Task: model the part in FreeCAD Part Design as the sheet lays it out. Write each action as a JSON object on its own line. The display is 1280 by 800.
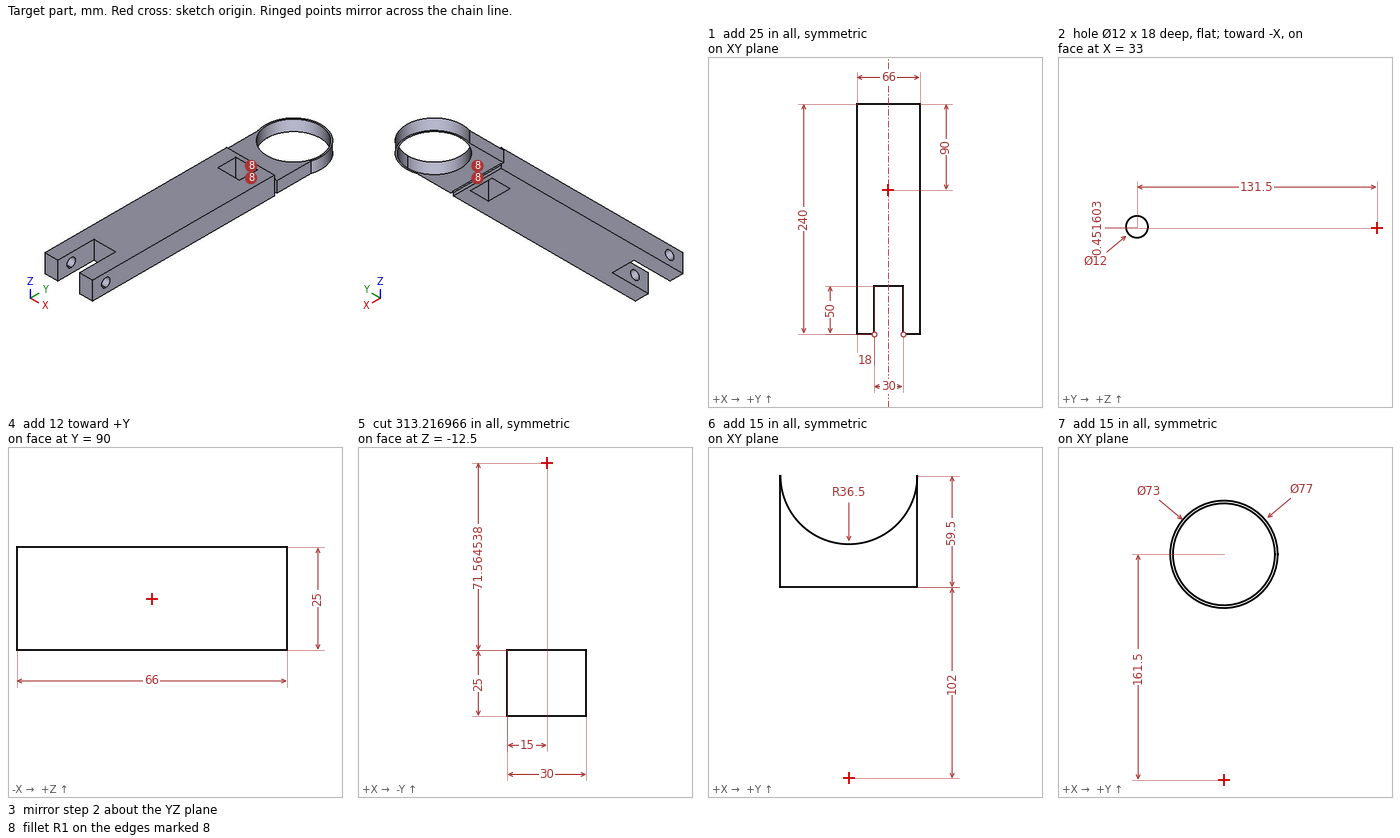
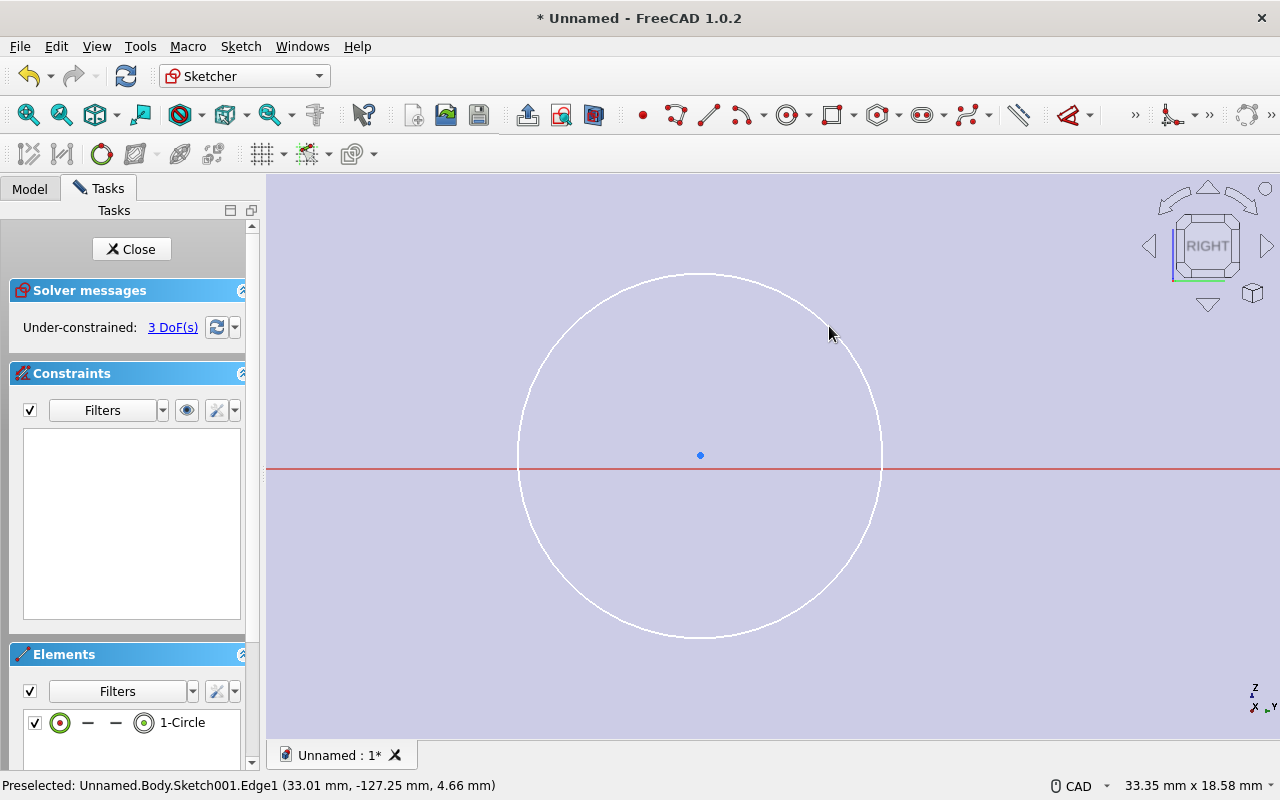
{"action": "left_click", "coordinate": [1068, 116]}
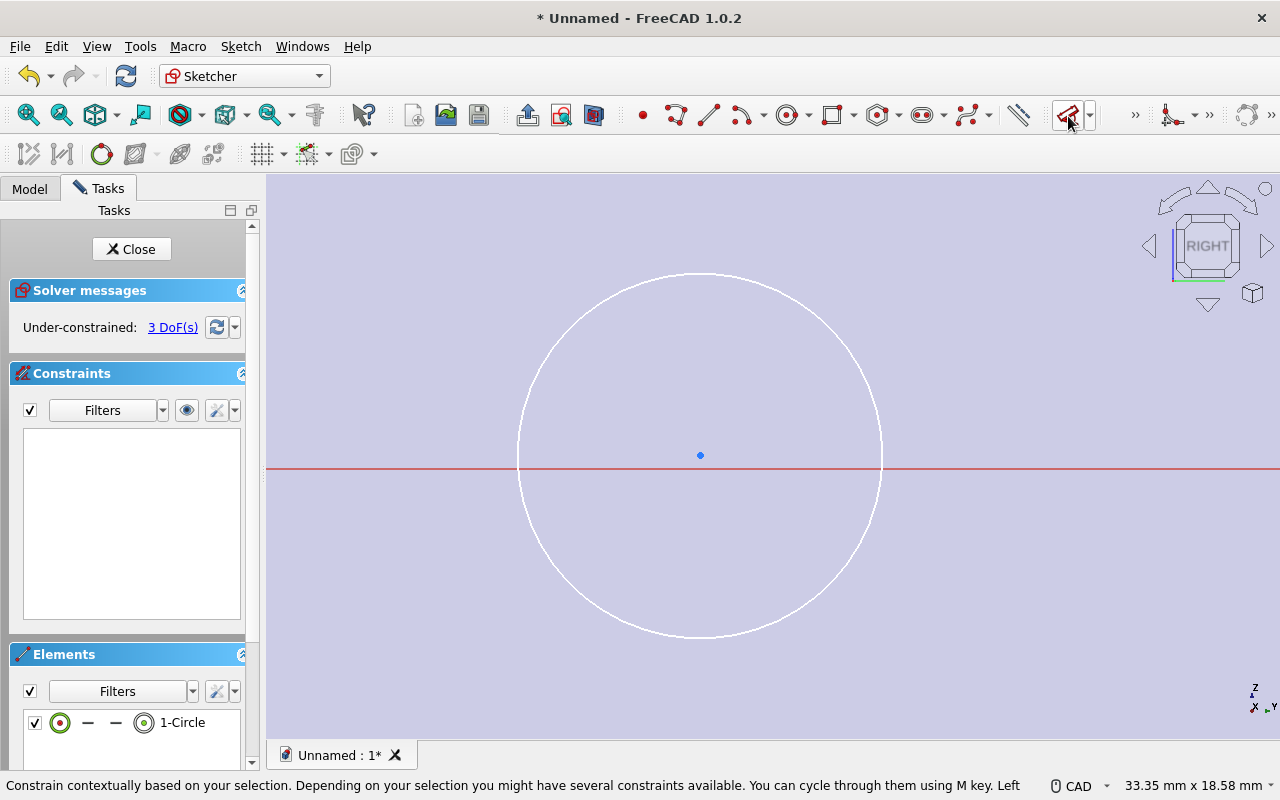
{"action": "left_click", "coordinate": [829, 327]}
{"action": "left_click", "coordinate": [852, 304]}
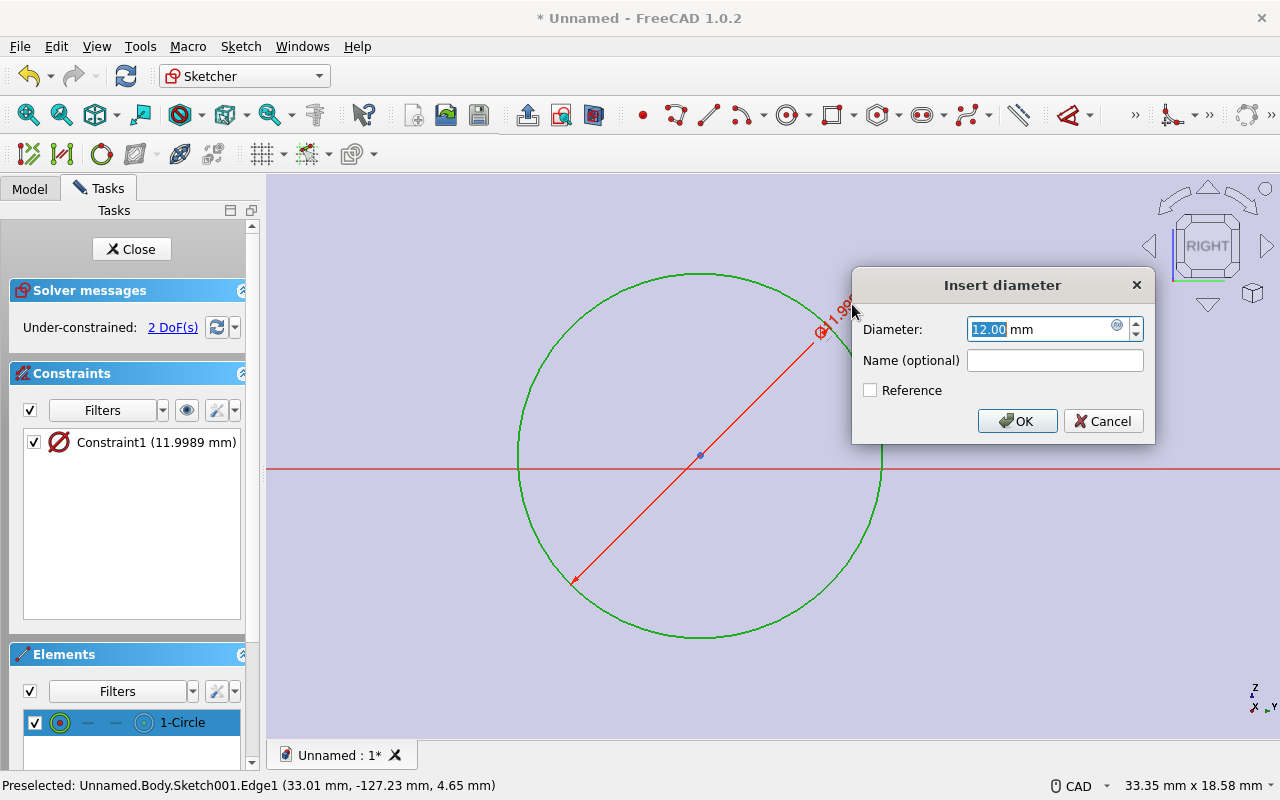
{"action": "type", "text": "12"}
{"action": "key", "text": "Return"}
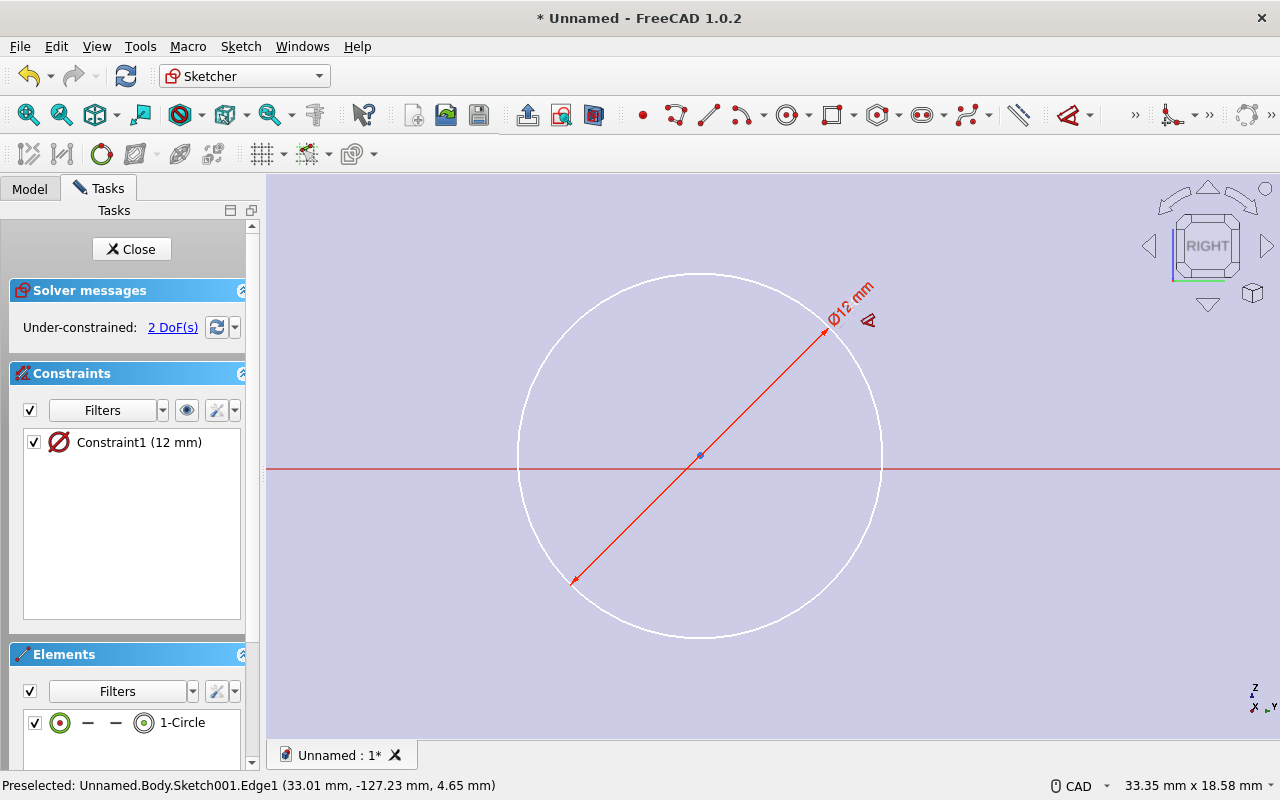
{"action": "left_click", "coordinate": [700, 456]}
{"action": "left_click", "coordinate": [908, 503]}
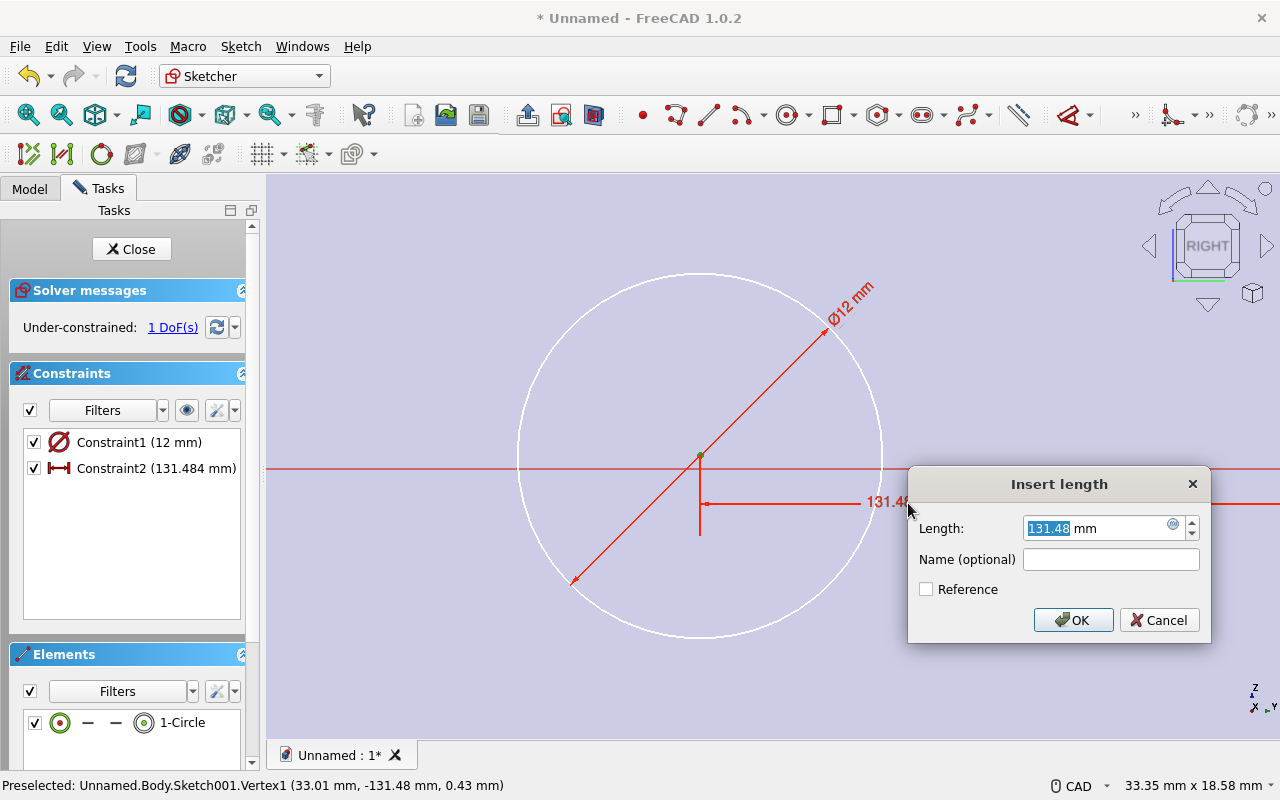
{"action": "type", "text": "131.5"}
{"action": "key", "text": "Return"}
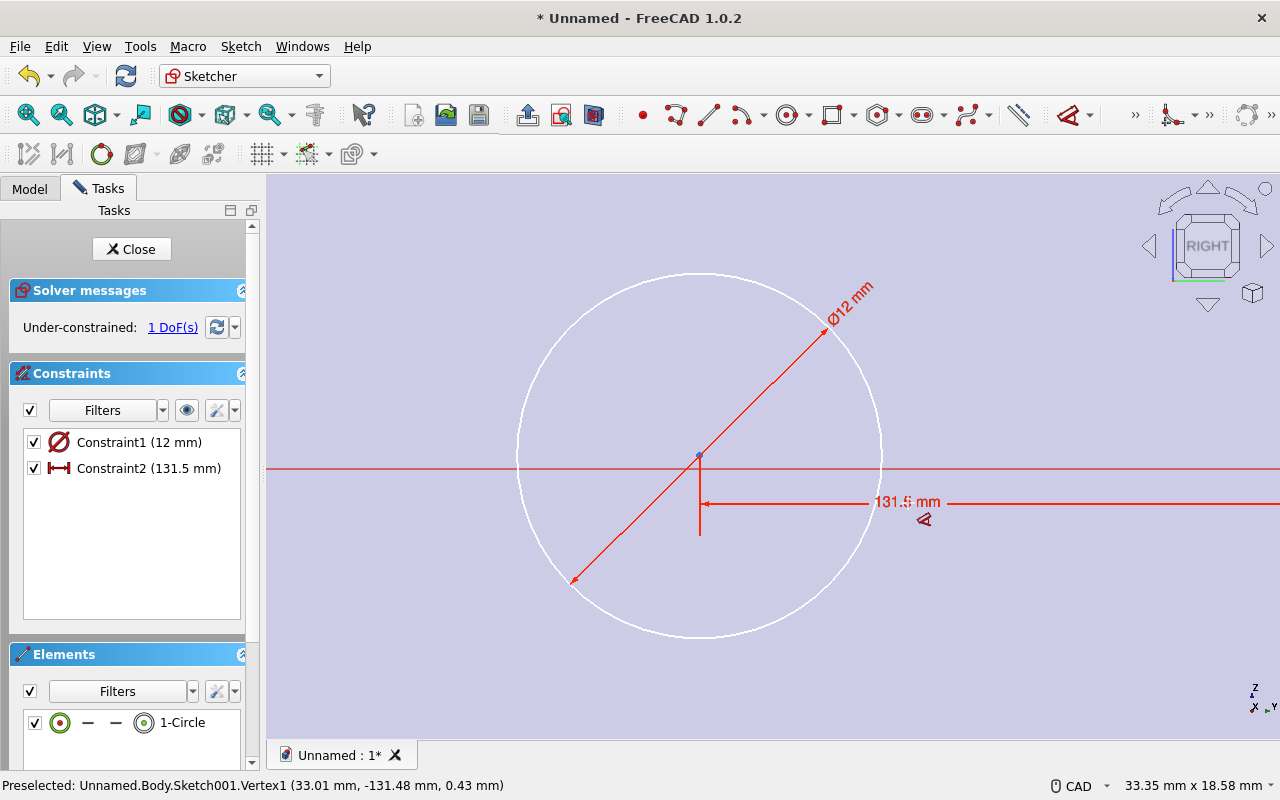
{"action": "scroll", "coordinate": [700, 456], "scroll_direction": "up", "scroll_amount": 6}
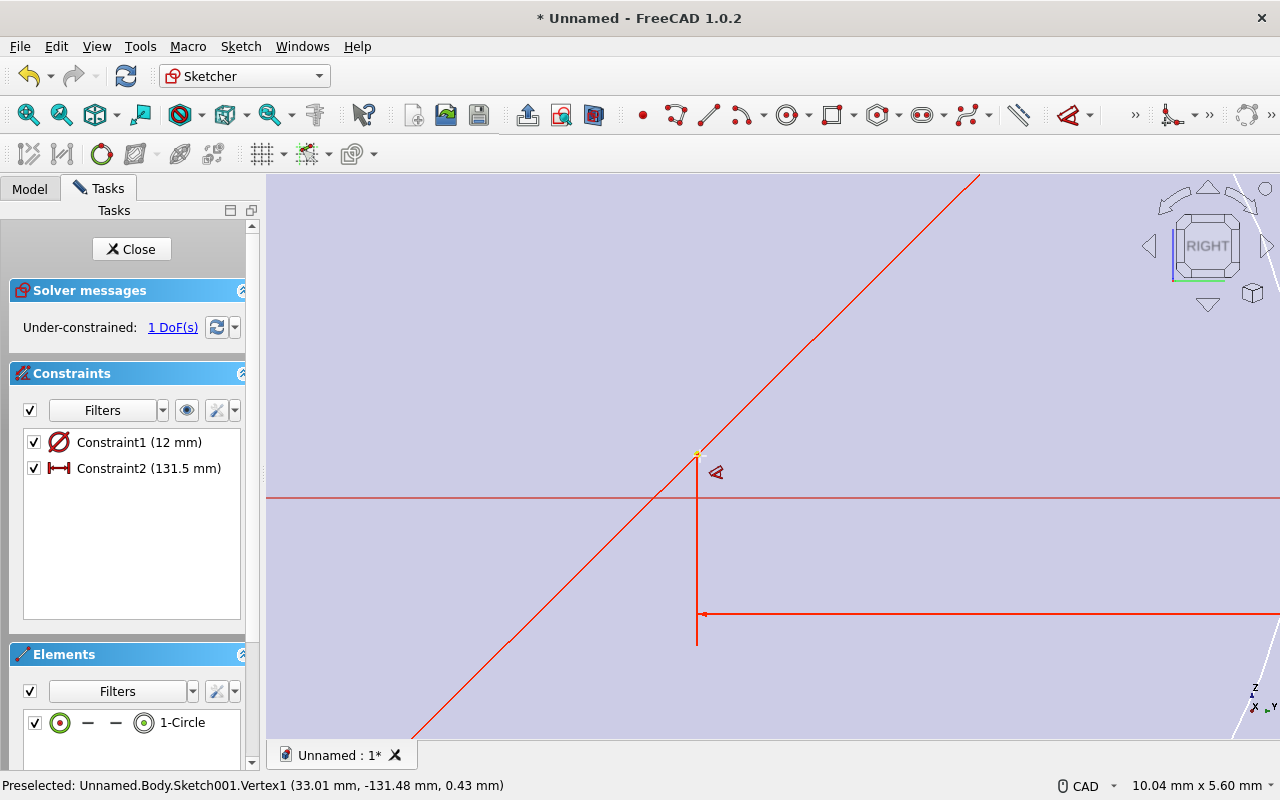
{"action": "left_click", "coordinate": [697, 455]}
{"action": "left_click", "coordinate": [663, 476]}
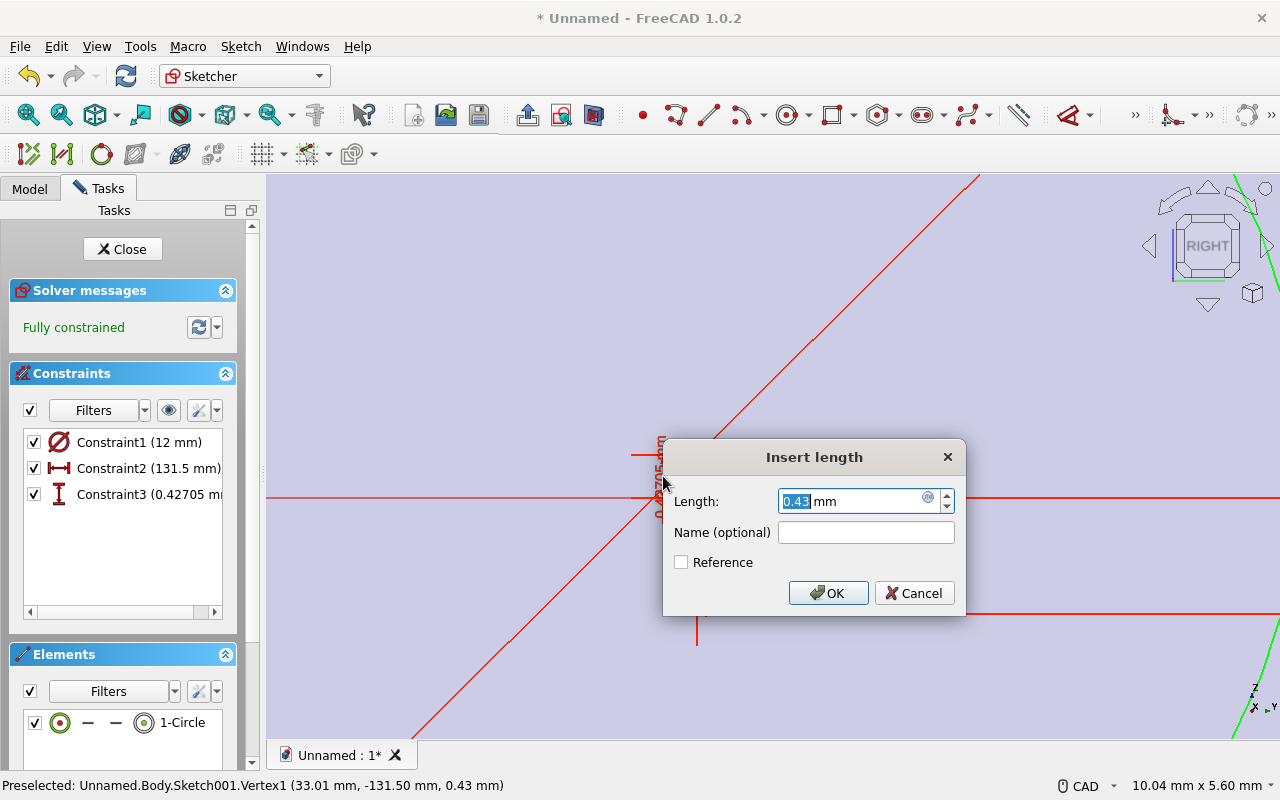
{"action": "type", "text": "0.451603"}
{"action": "key", "text": "Return"}
{"action": "key", "text": "Escape"}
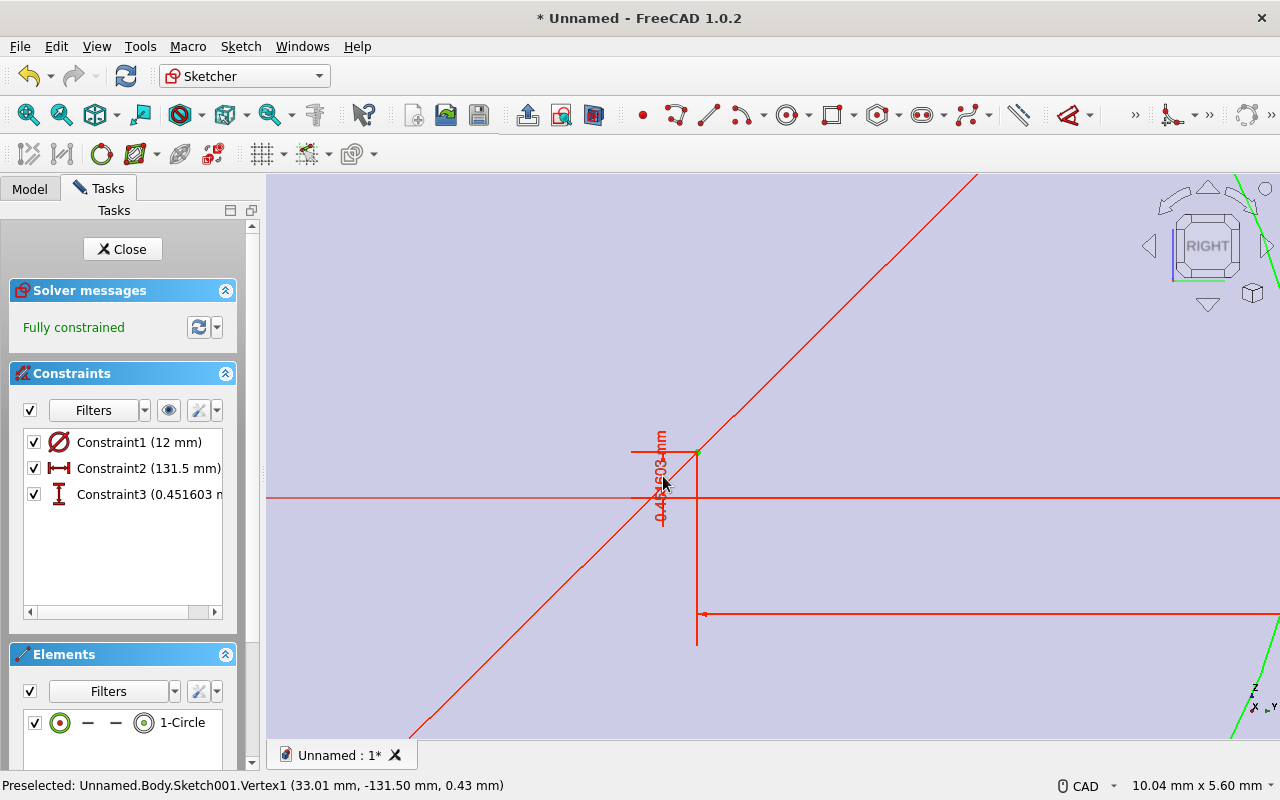
{"action": "left_click", "coordinate": [123, 249]}